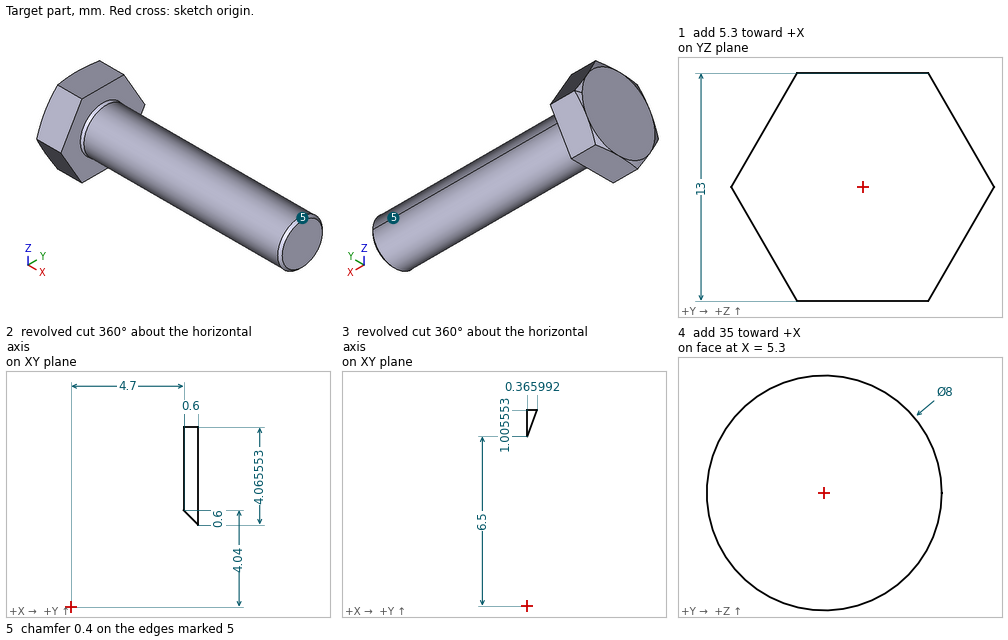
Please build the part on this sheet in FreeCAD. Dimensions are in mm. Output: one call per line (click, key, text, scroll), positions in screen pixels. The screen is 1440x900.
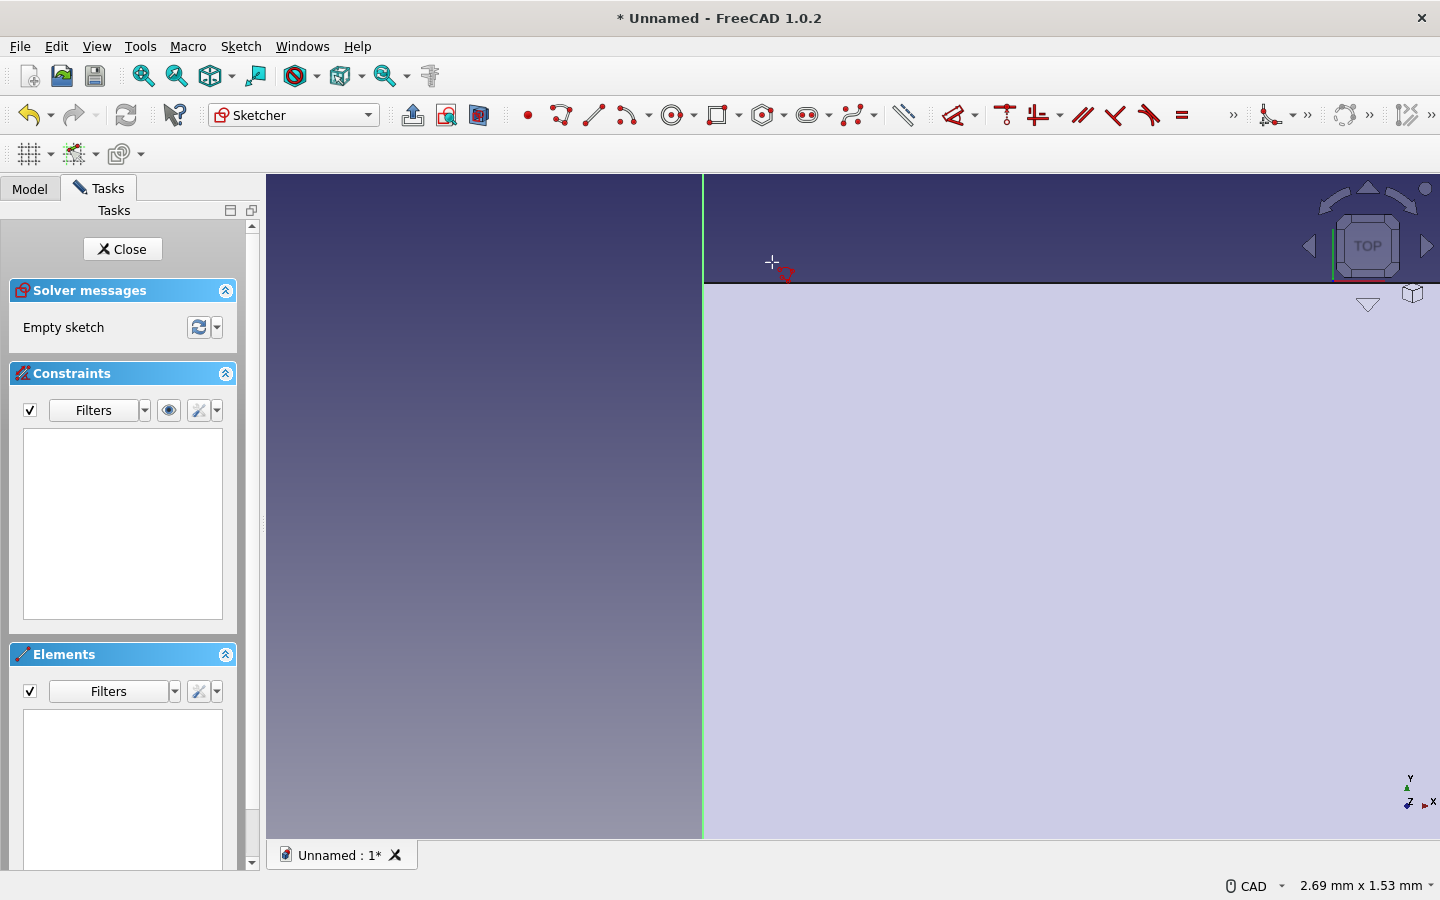
click(703, 721)
click(862, 283)
click(712, 283)
click(703, 722)
key(Escape)
key(Escape)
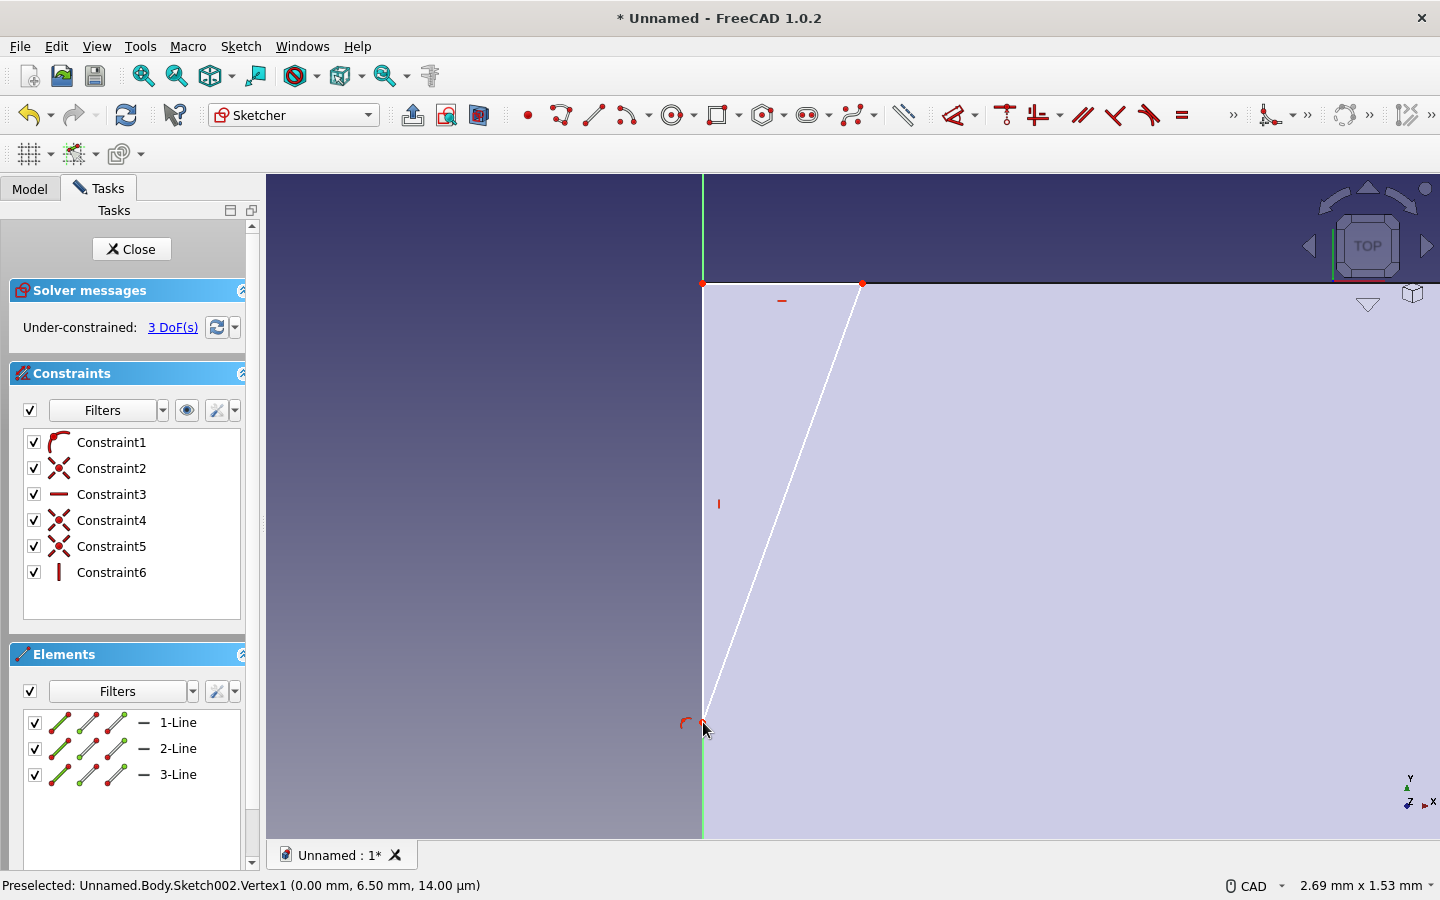
key(d)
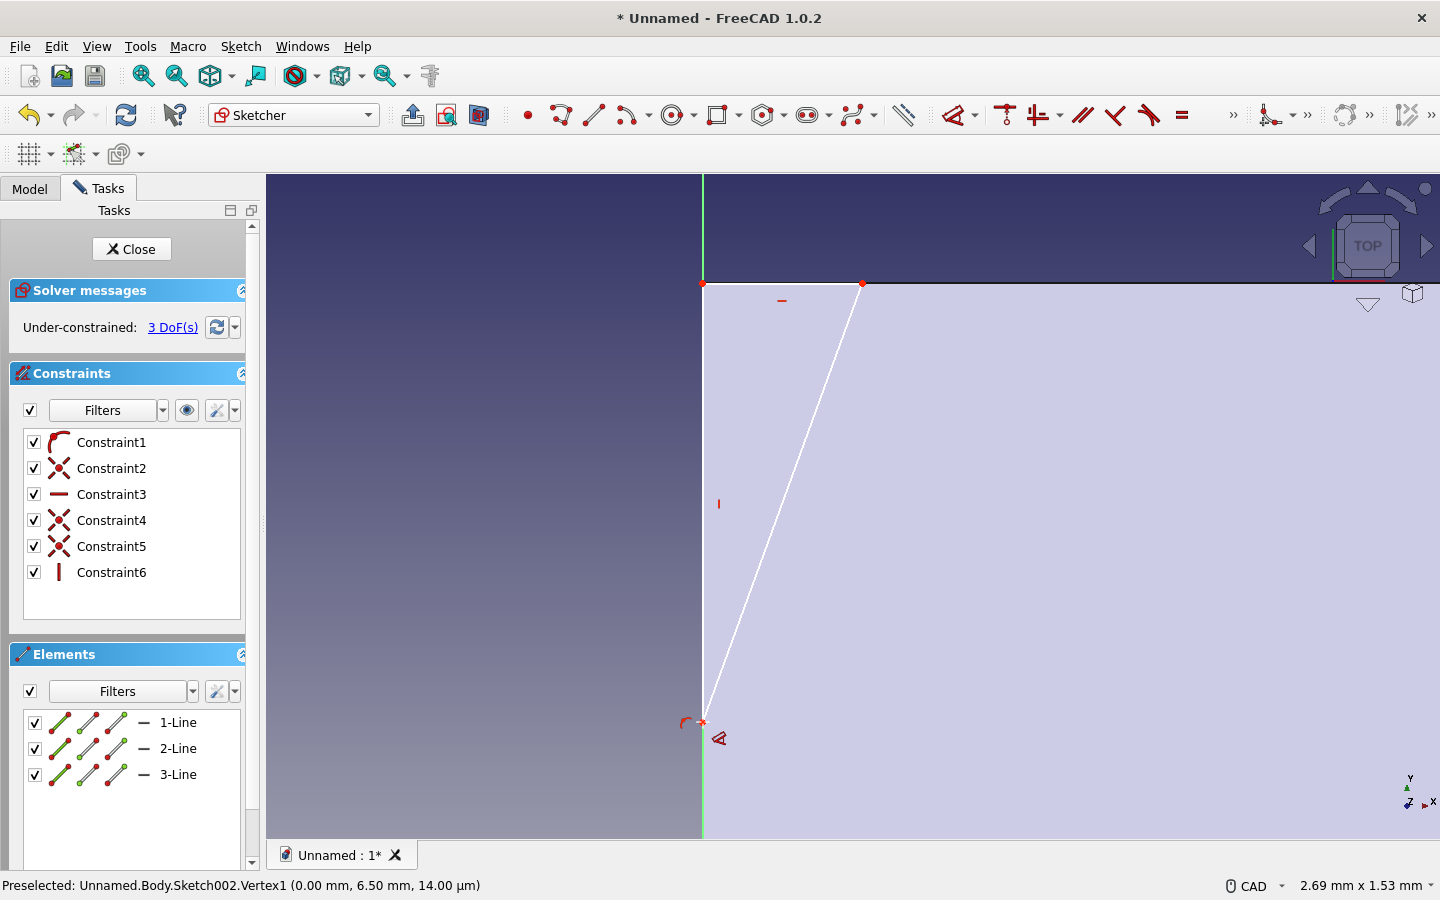
click(703, 722)
click(669, 767)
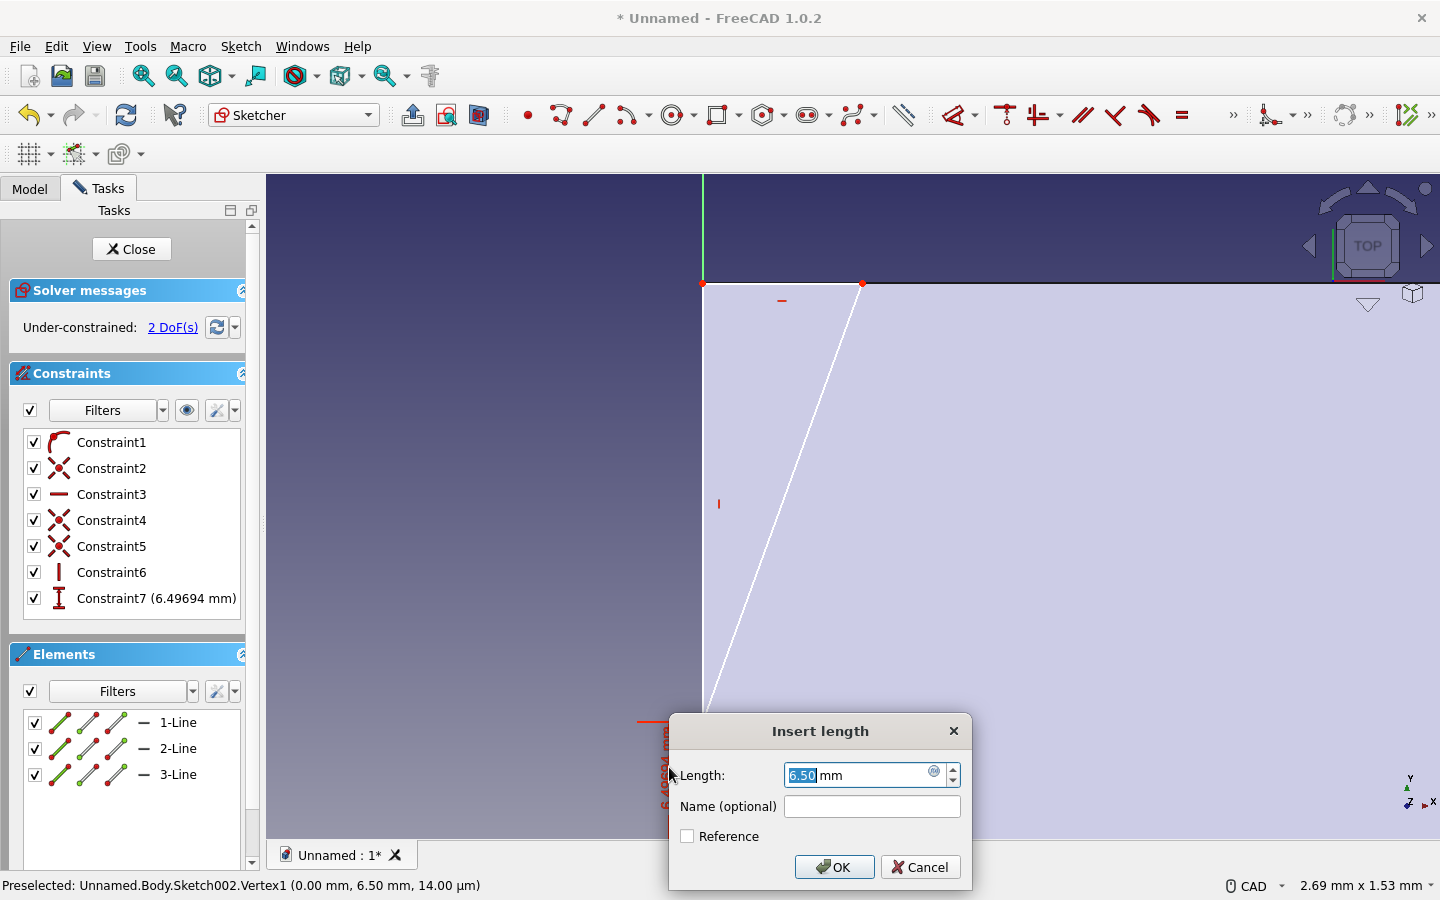
text(6.5)
key(Return)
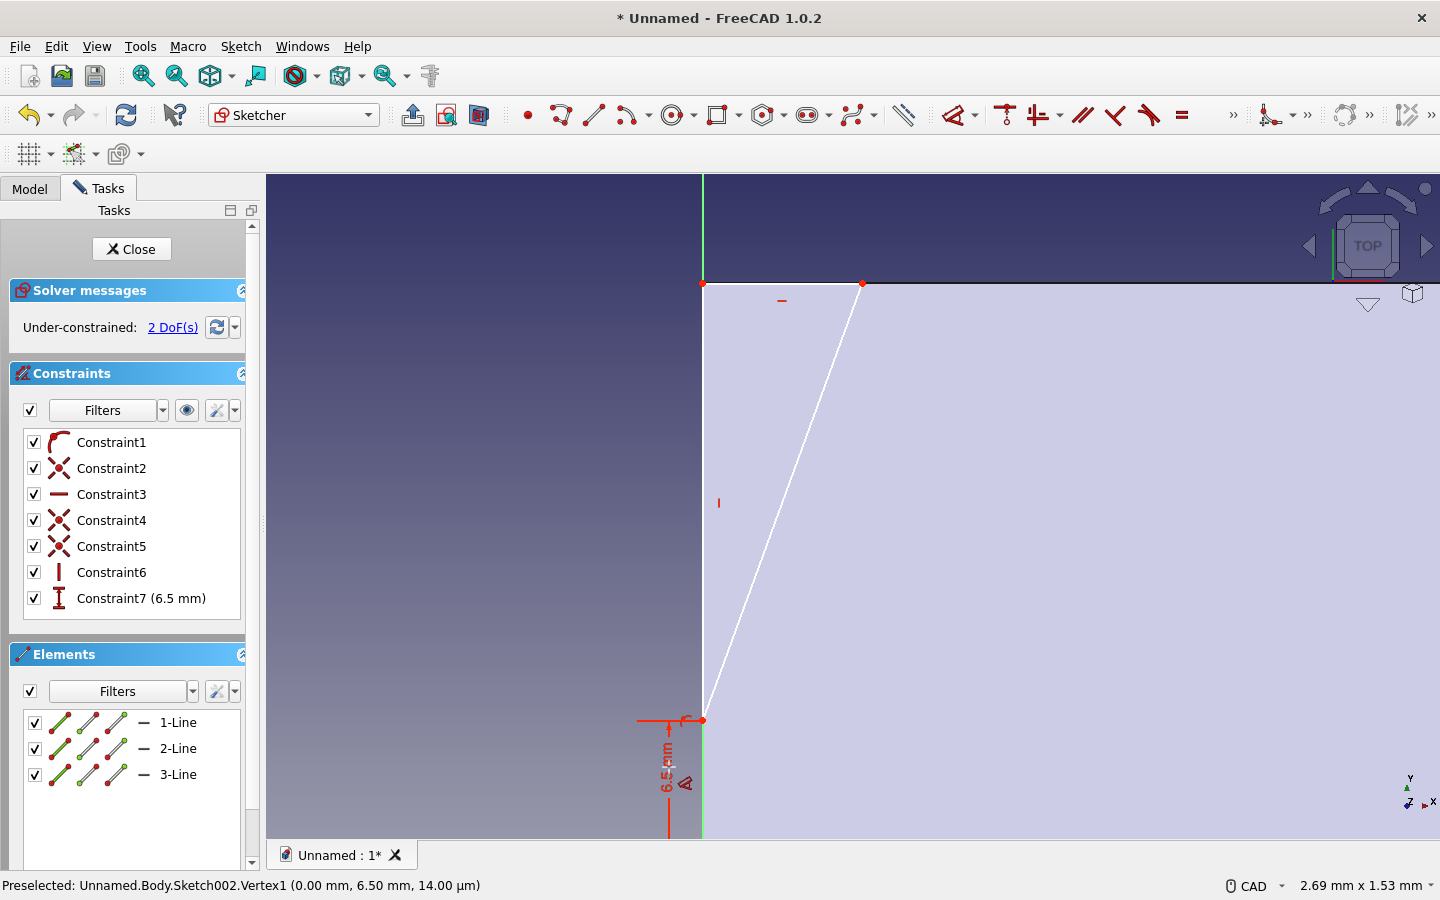
click(814, 284)
click(782, 250)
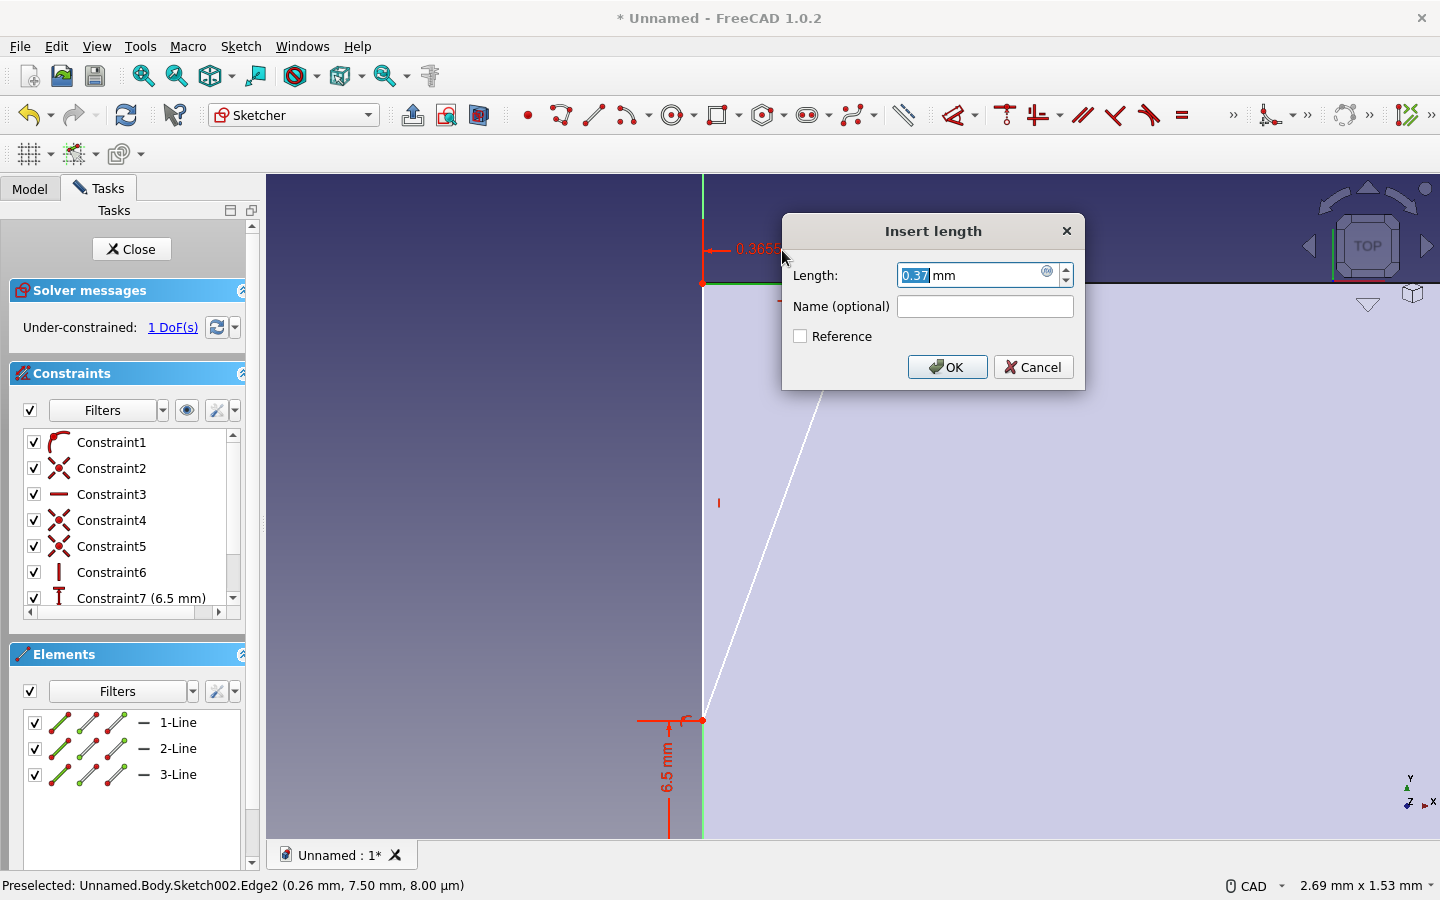
text(0.365992)
key(Return)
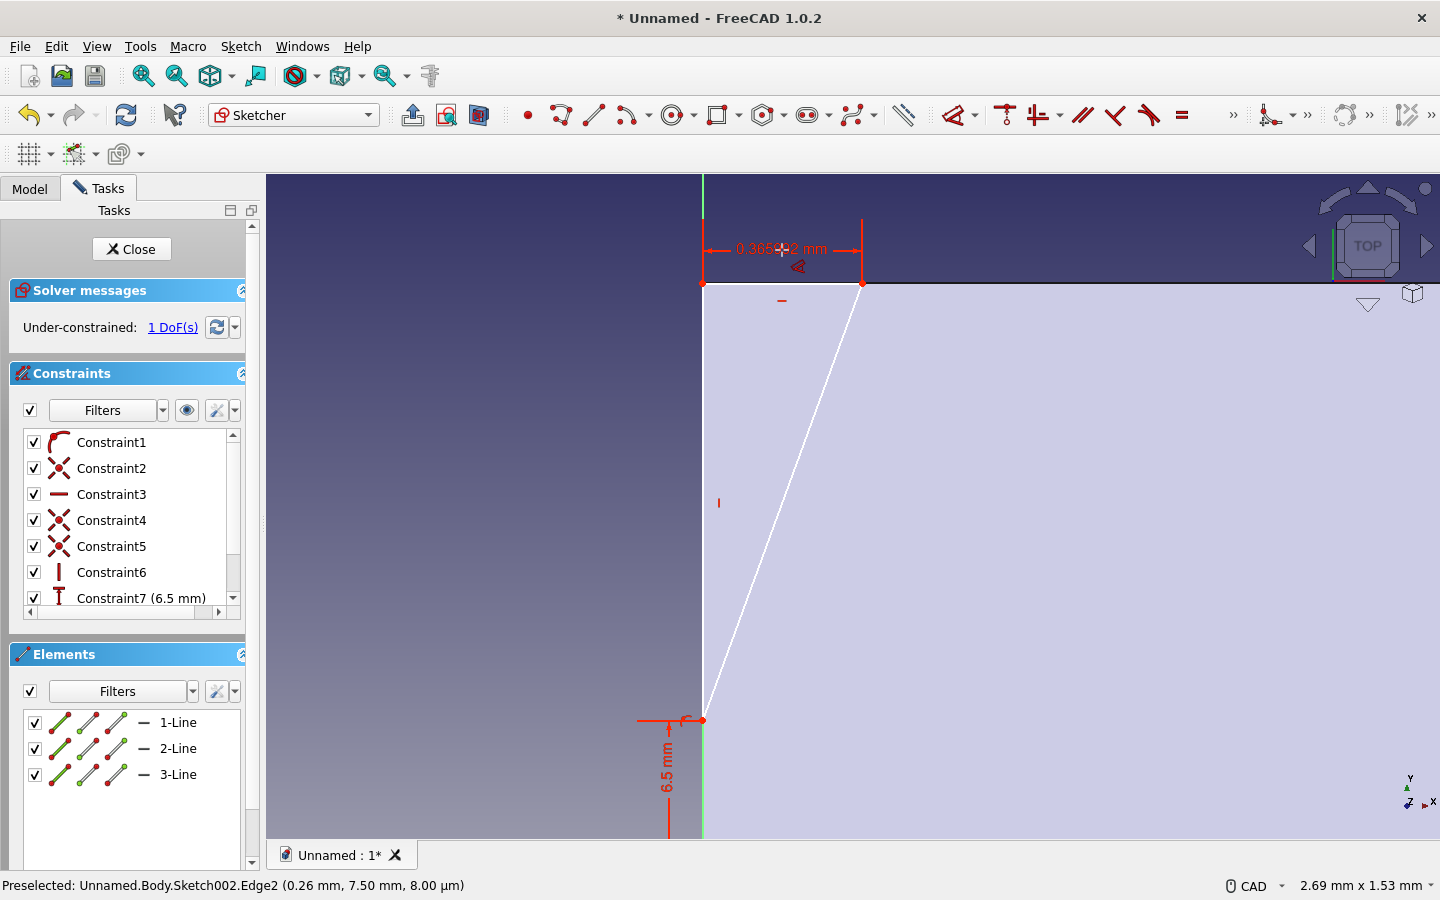
click(703, 415)
click(669, 502)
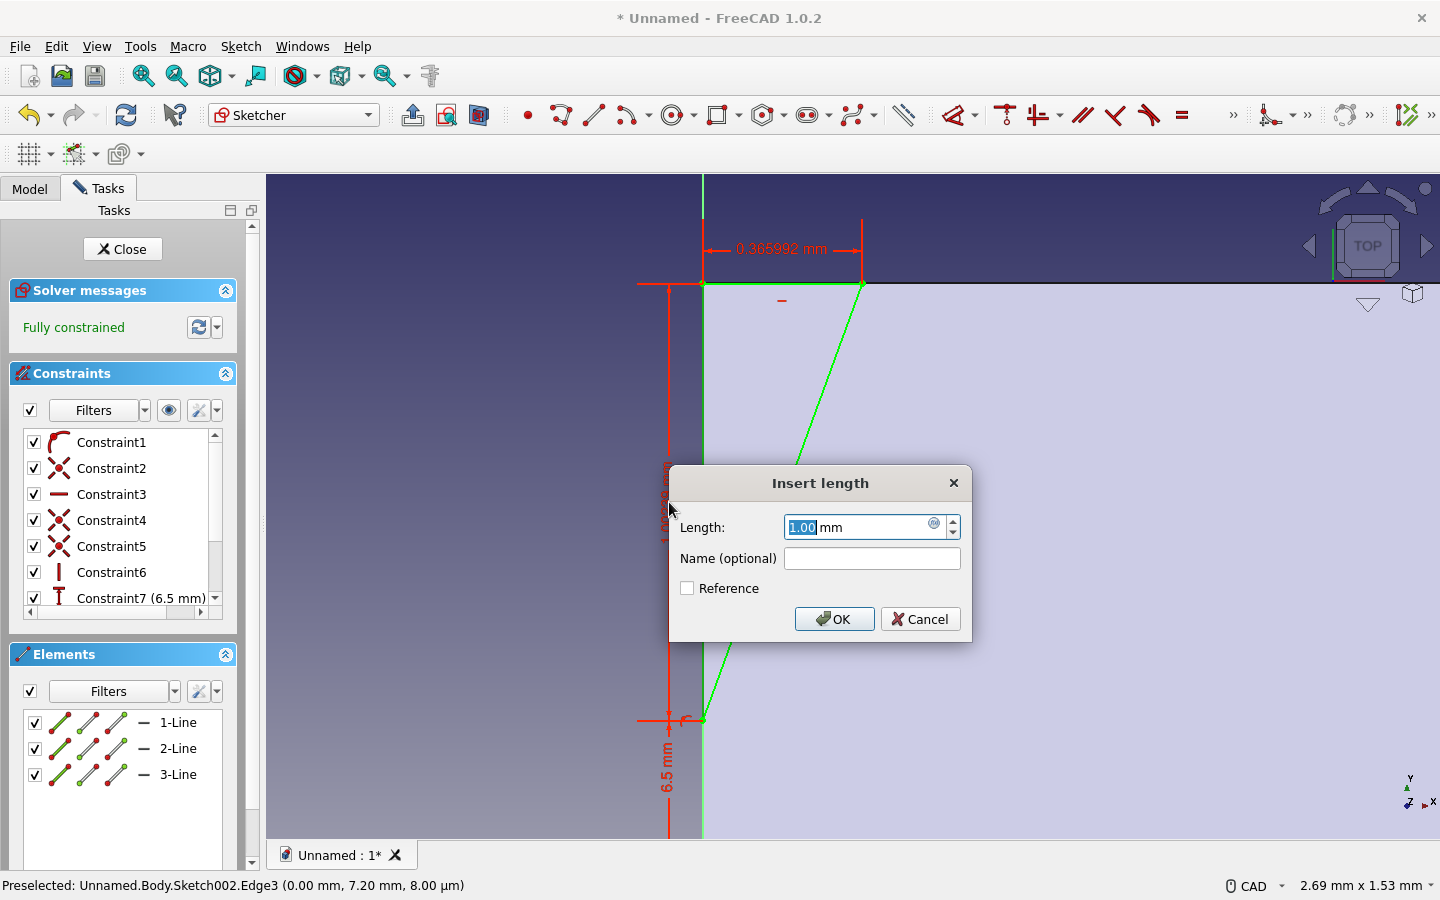
text(1.005553)
key(Return)
key(Escape)